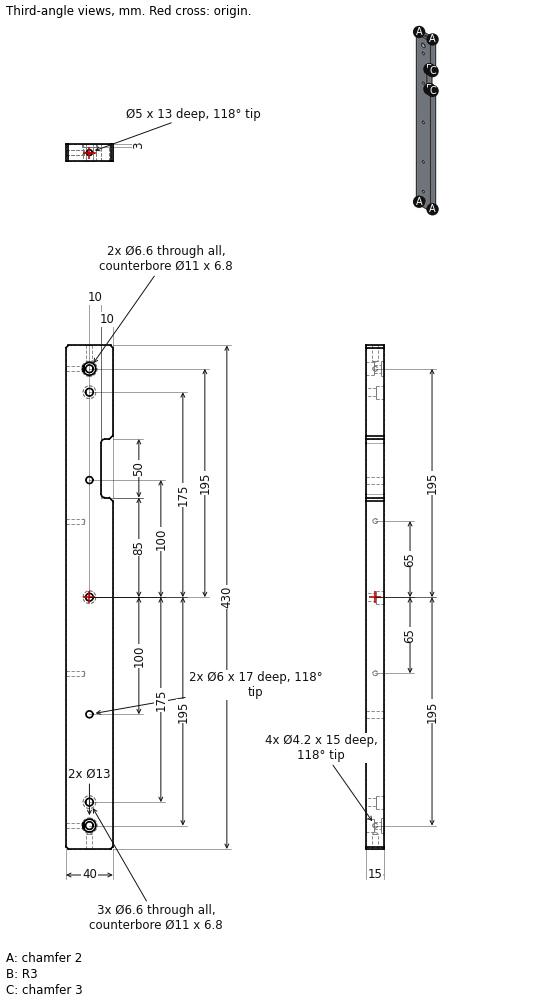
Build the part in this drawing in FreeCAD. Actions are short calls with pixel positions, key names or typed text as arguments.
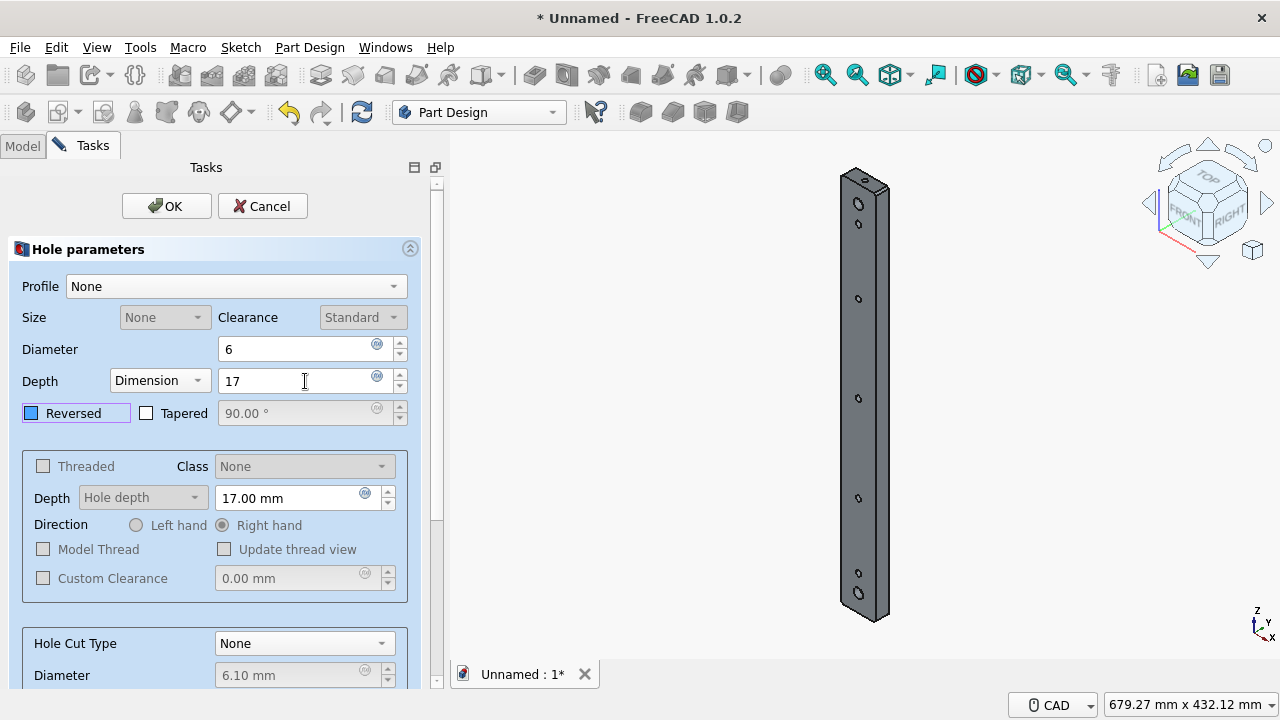
click(167, 206)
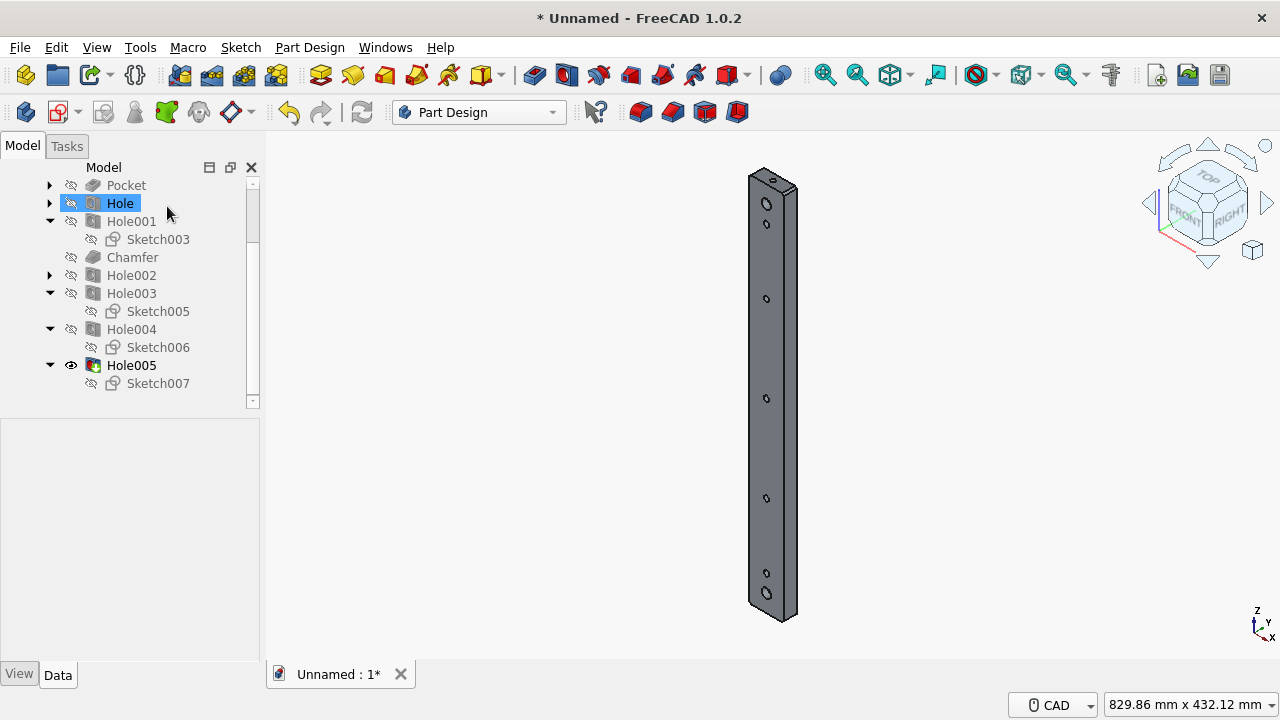
click(767, 336)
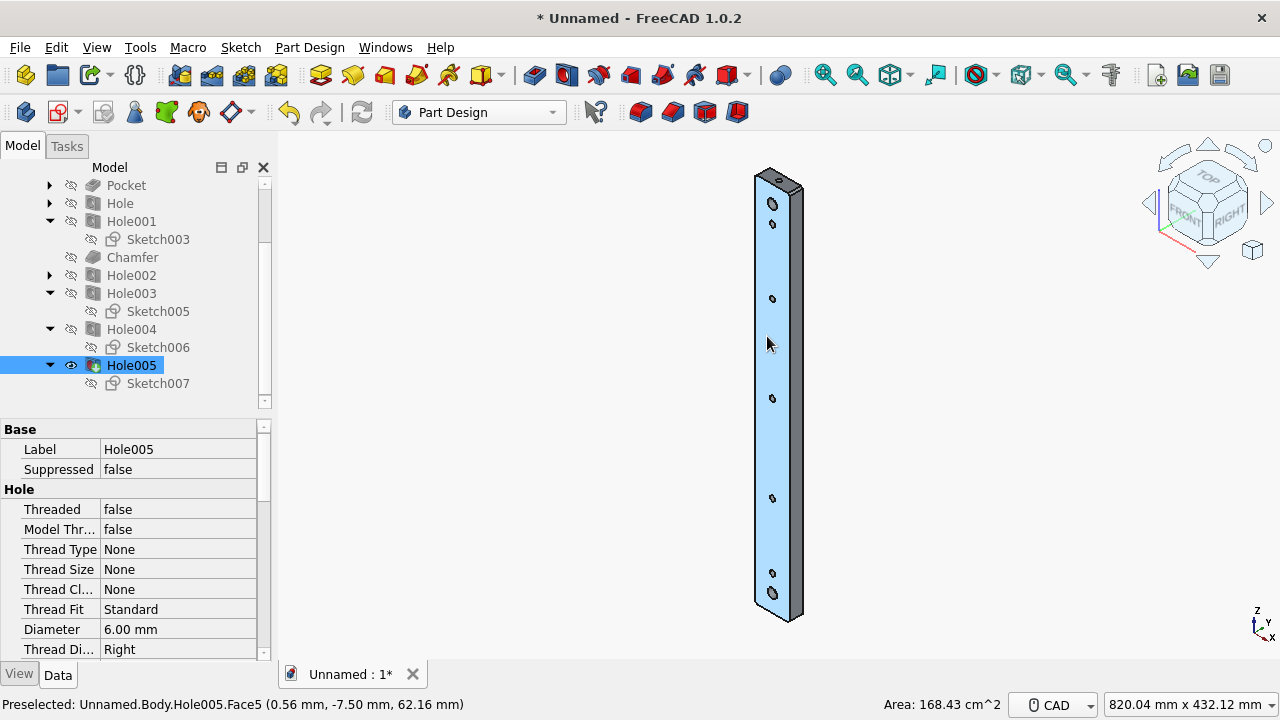
click(58, 112)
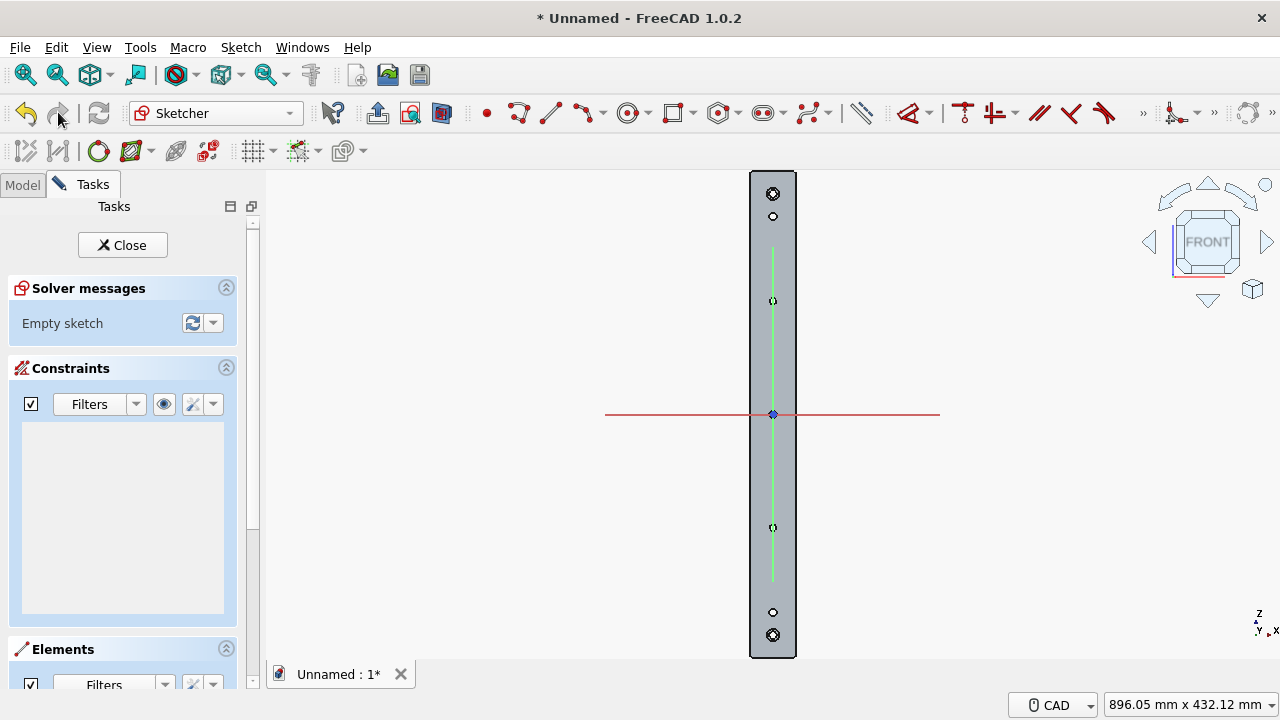
scroll(812, 259, up, 8)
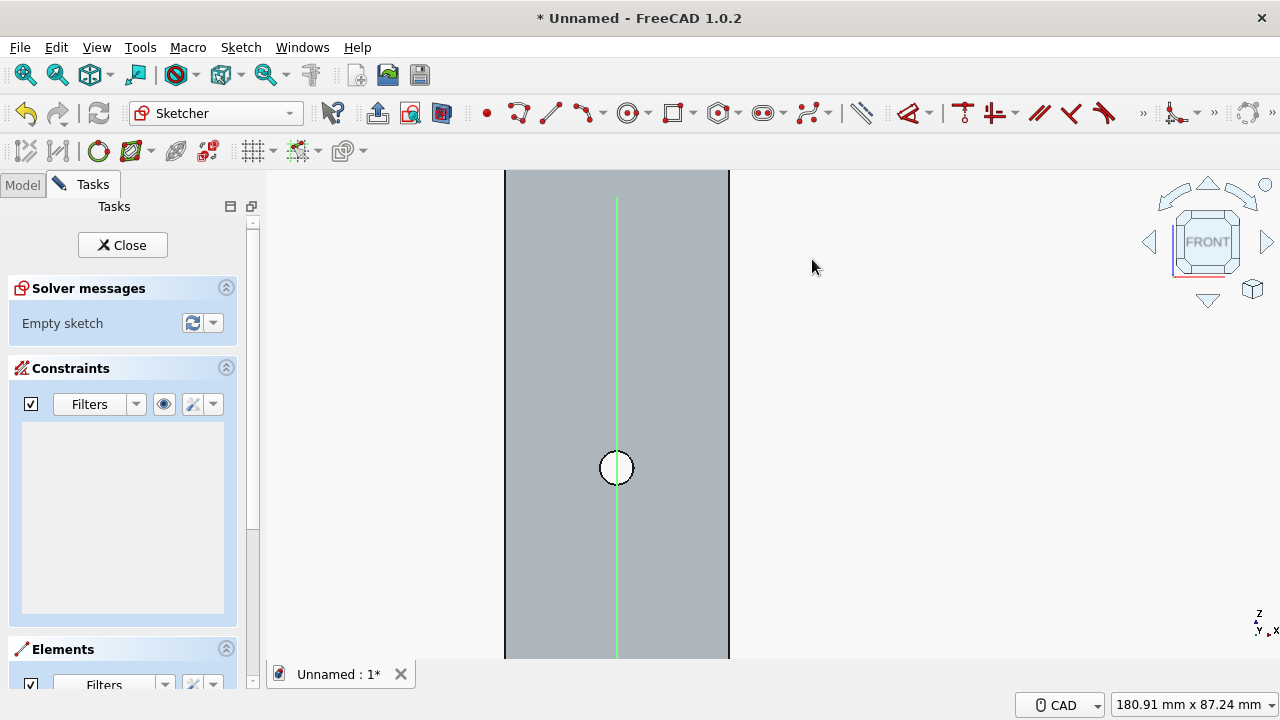
click(674, 114)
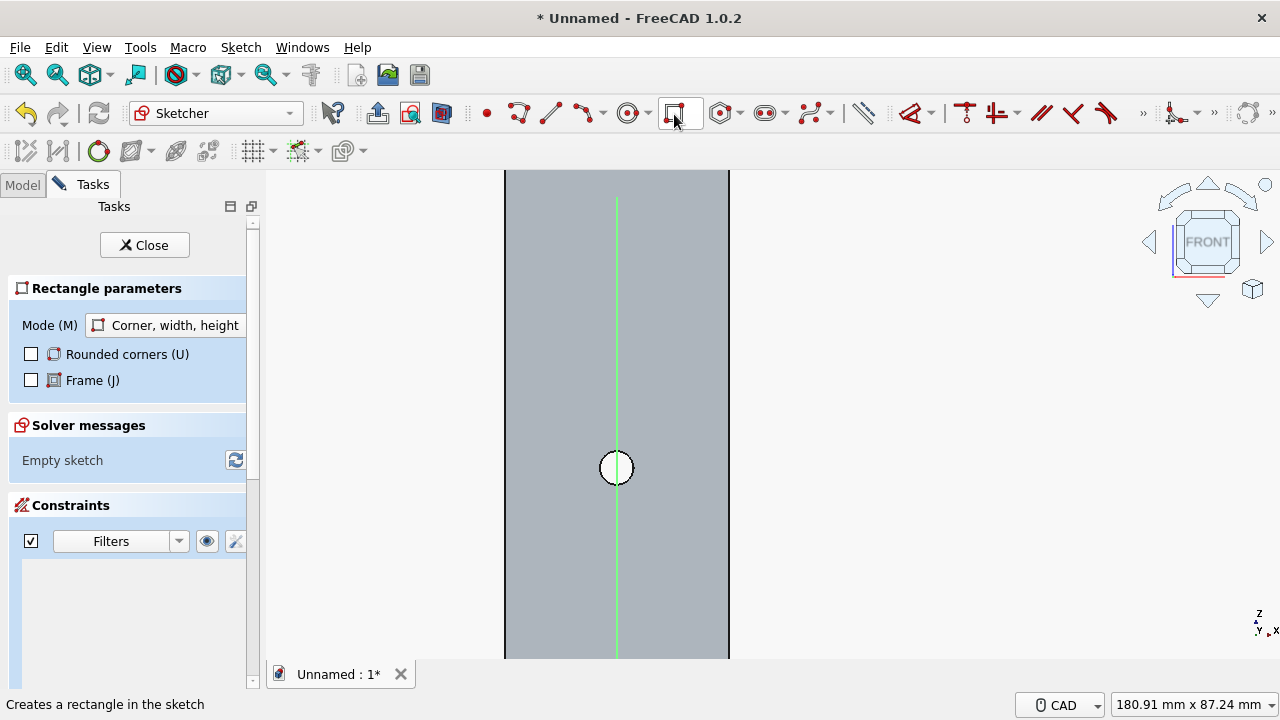
click(673, 272)
move(729, 552)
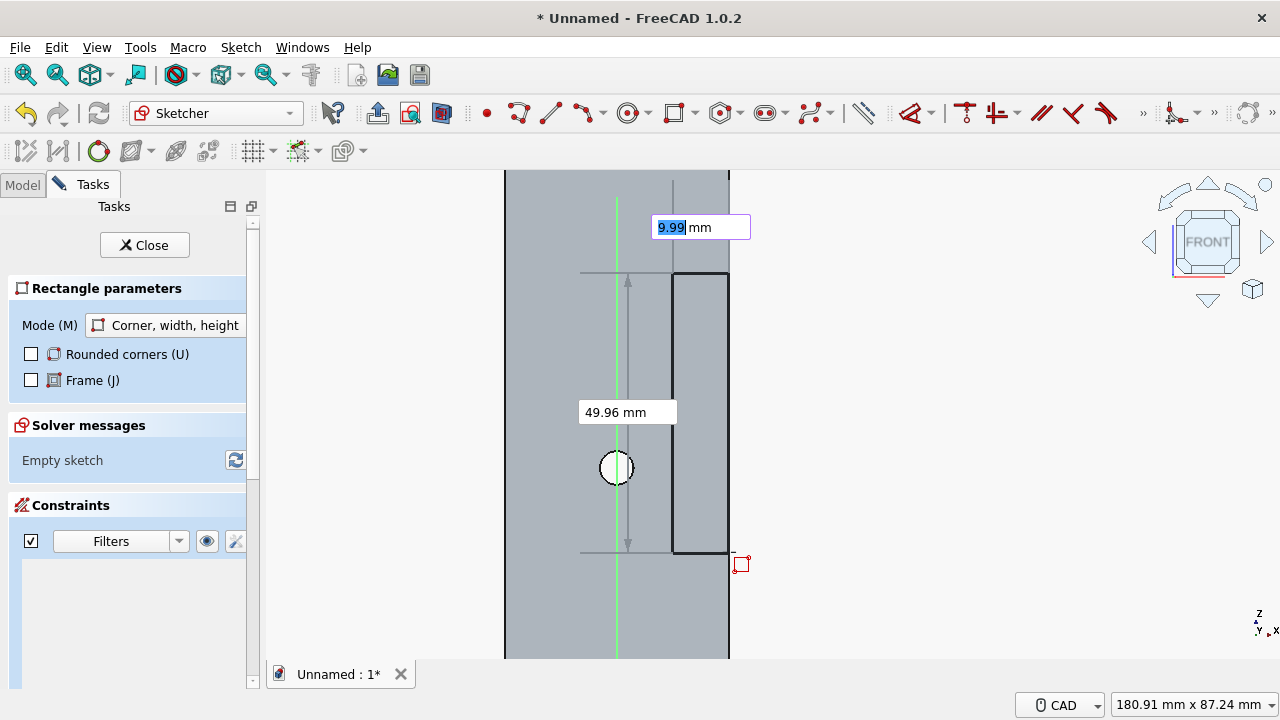
text(10)
key(Tab)
text(50)
key(Return)
key(Escape)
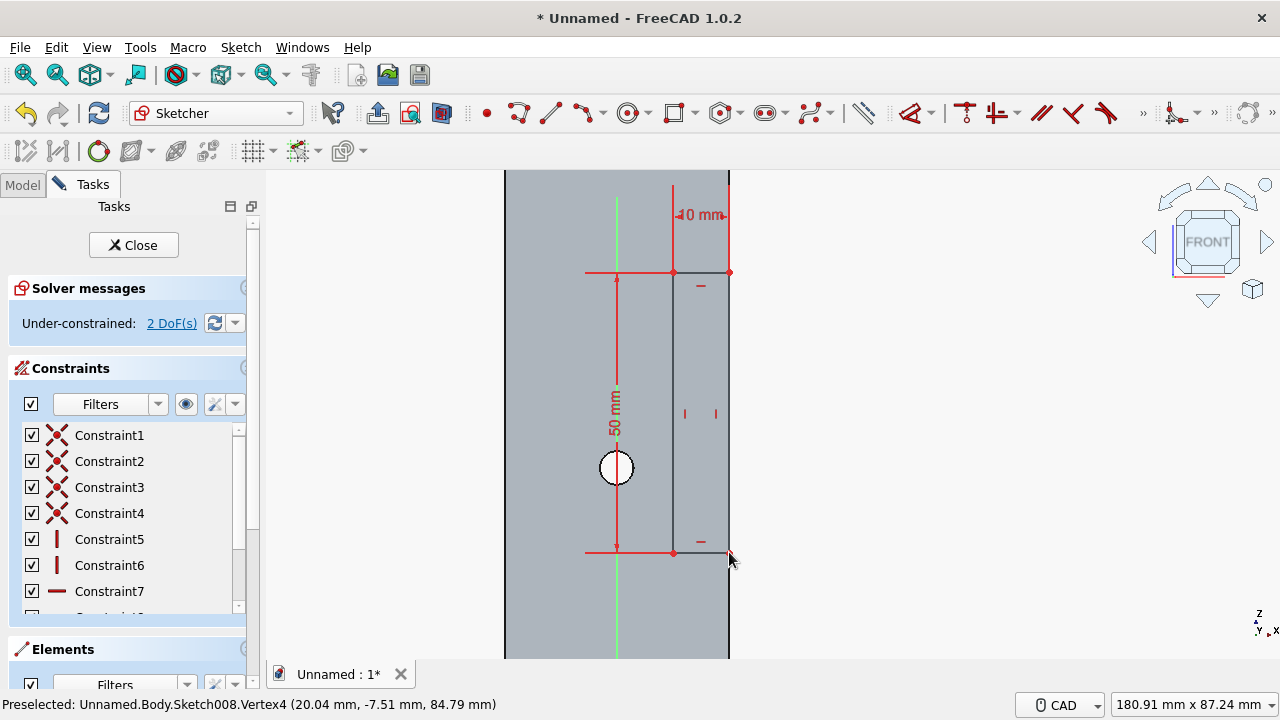
click(910, 114)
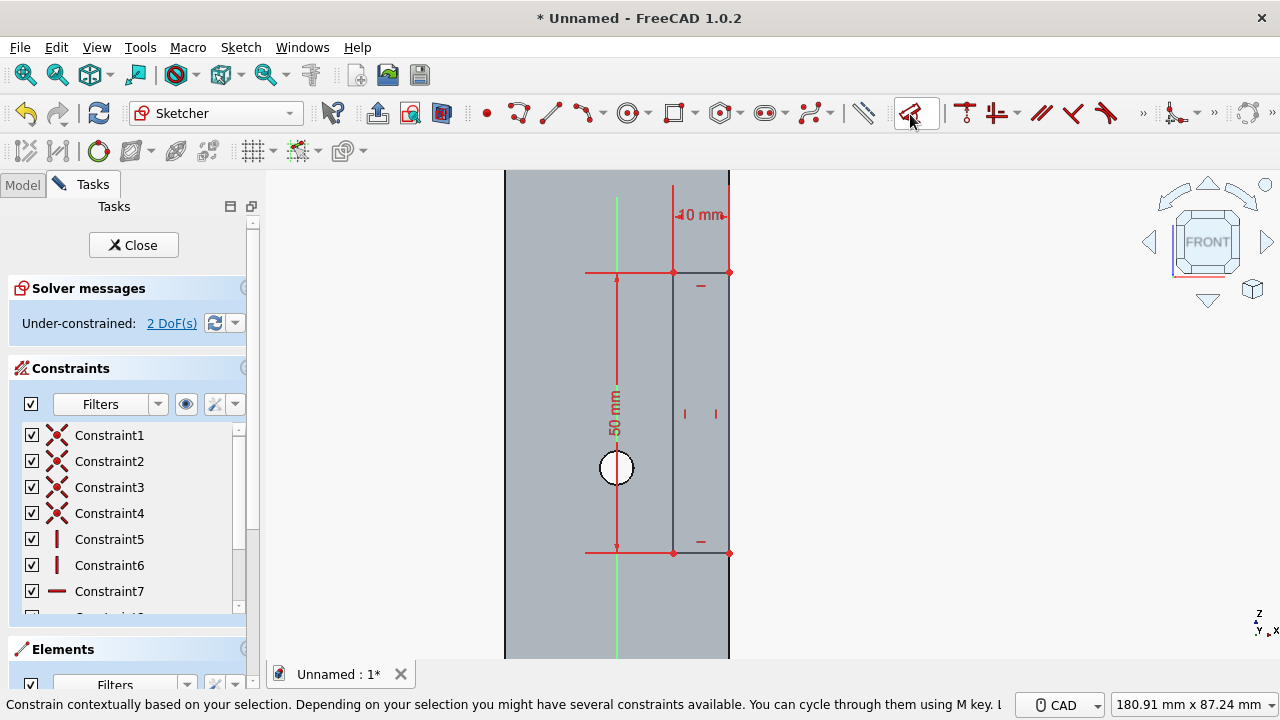
click(673, 273)
click(645, 239)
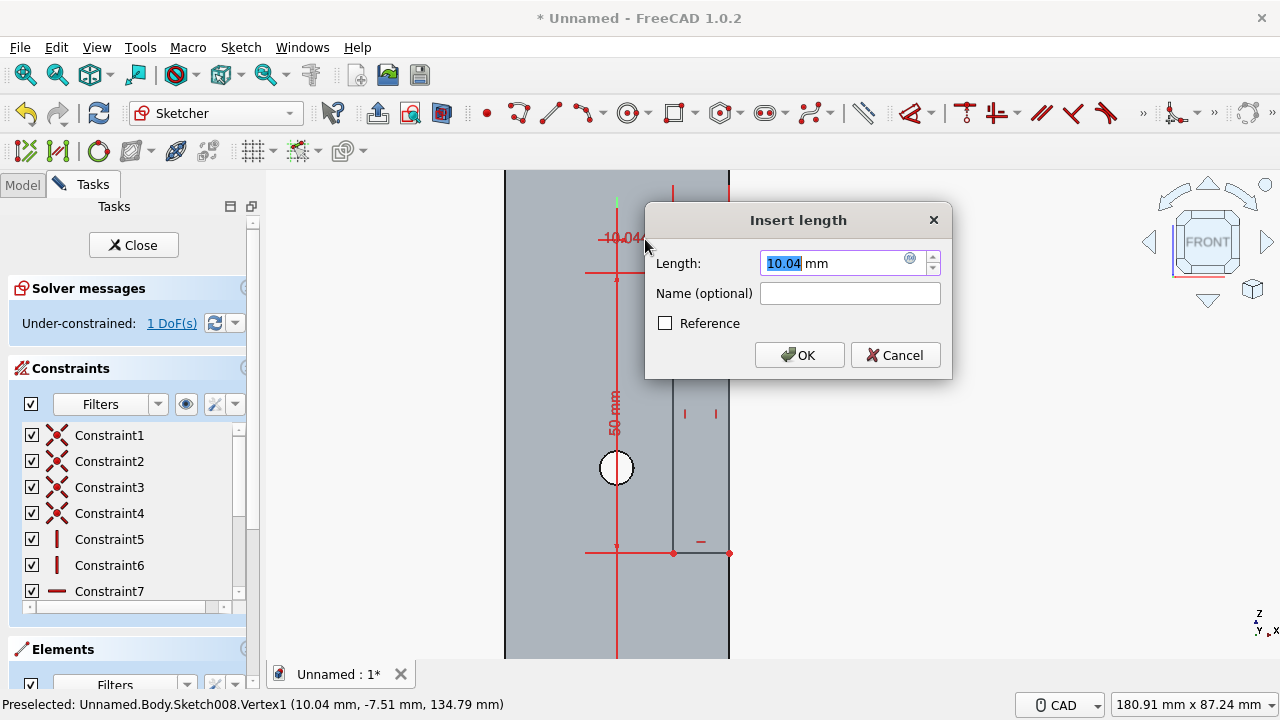
text(10)
key(Return)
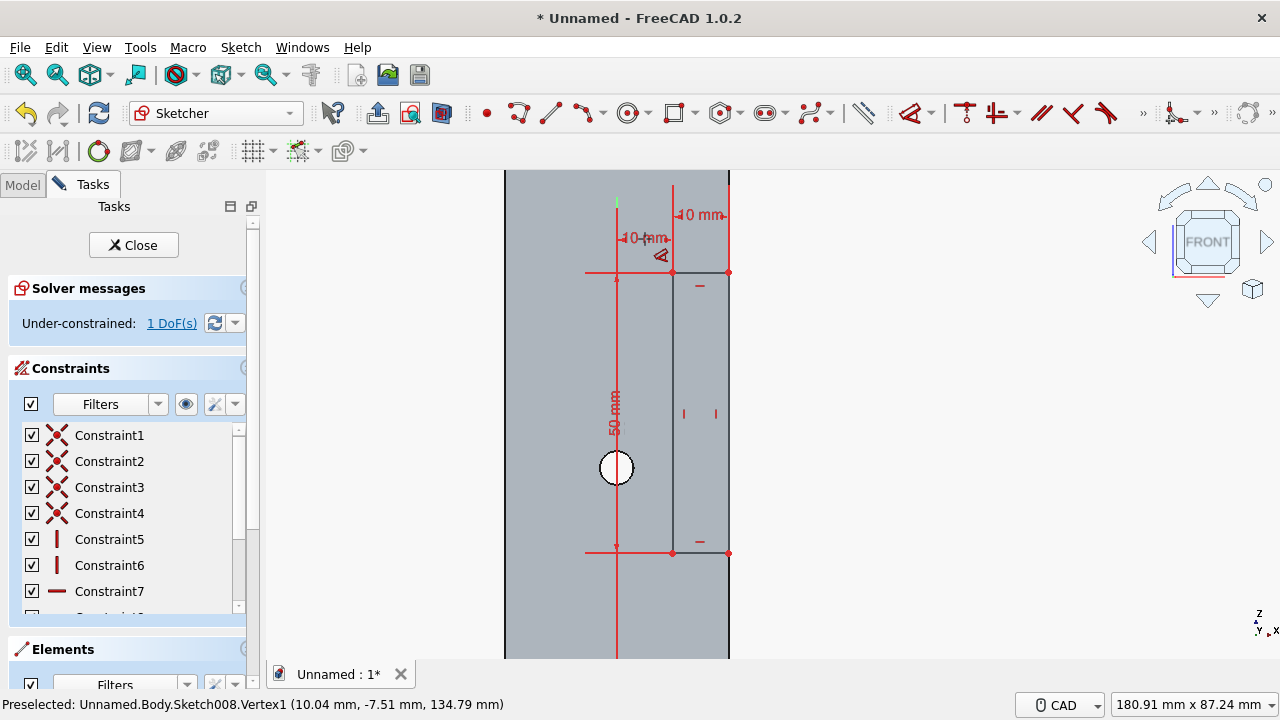
click(673, 553)
click(583, 592)